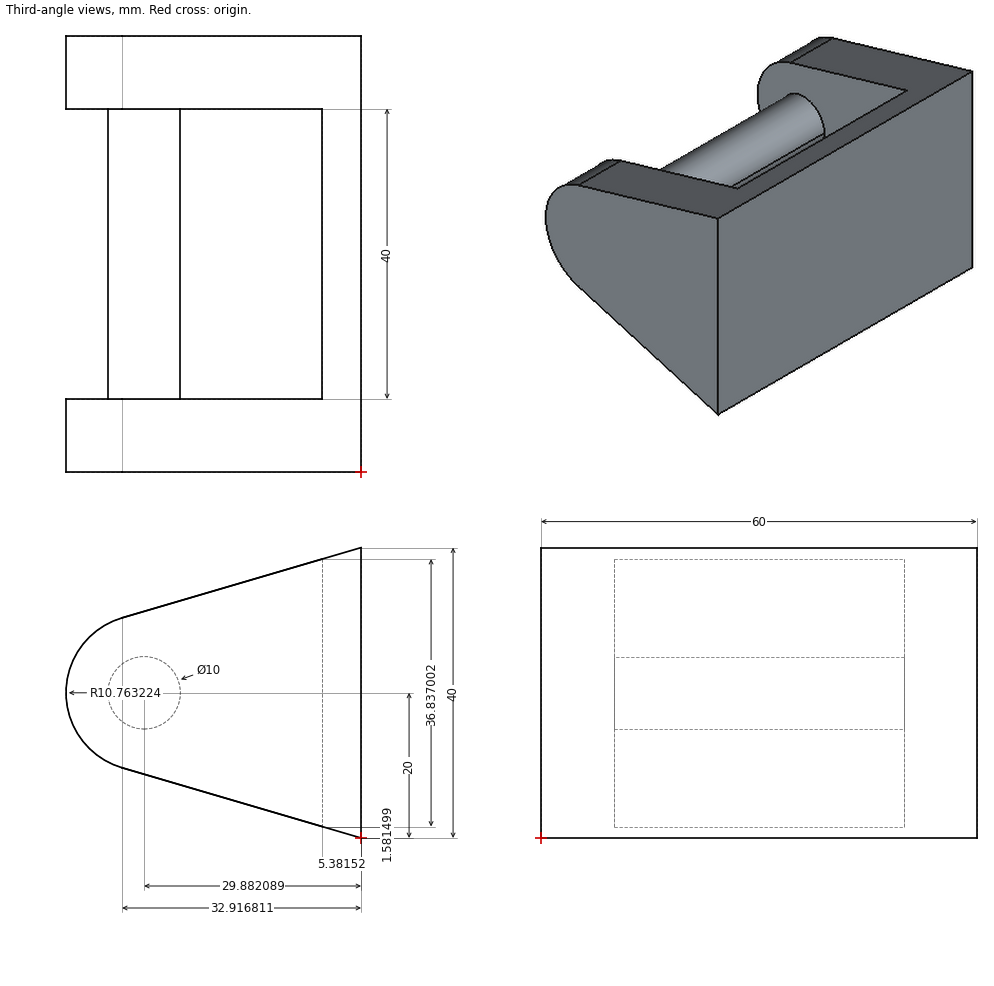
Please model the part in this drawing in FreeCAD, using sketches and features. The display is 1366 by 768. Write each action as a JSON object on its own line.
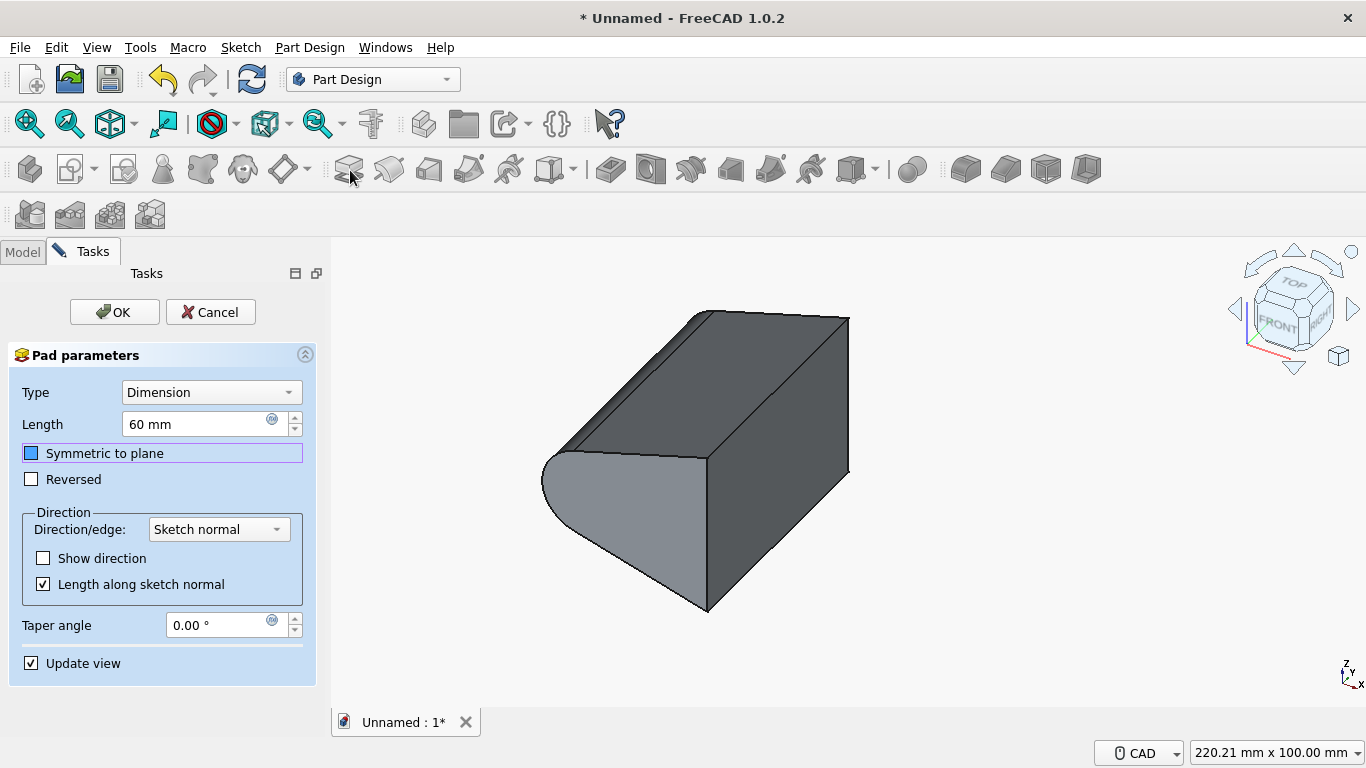
{"action": "left_click", "coordinate": [30, 479]}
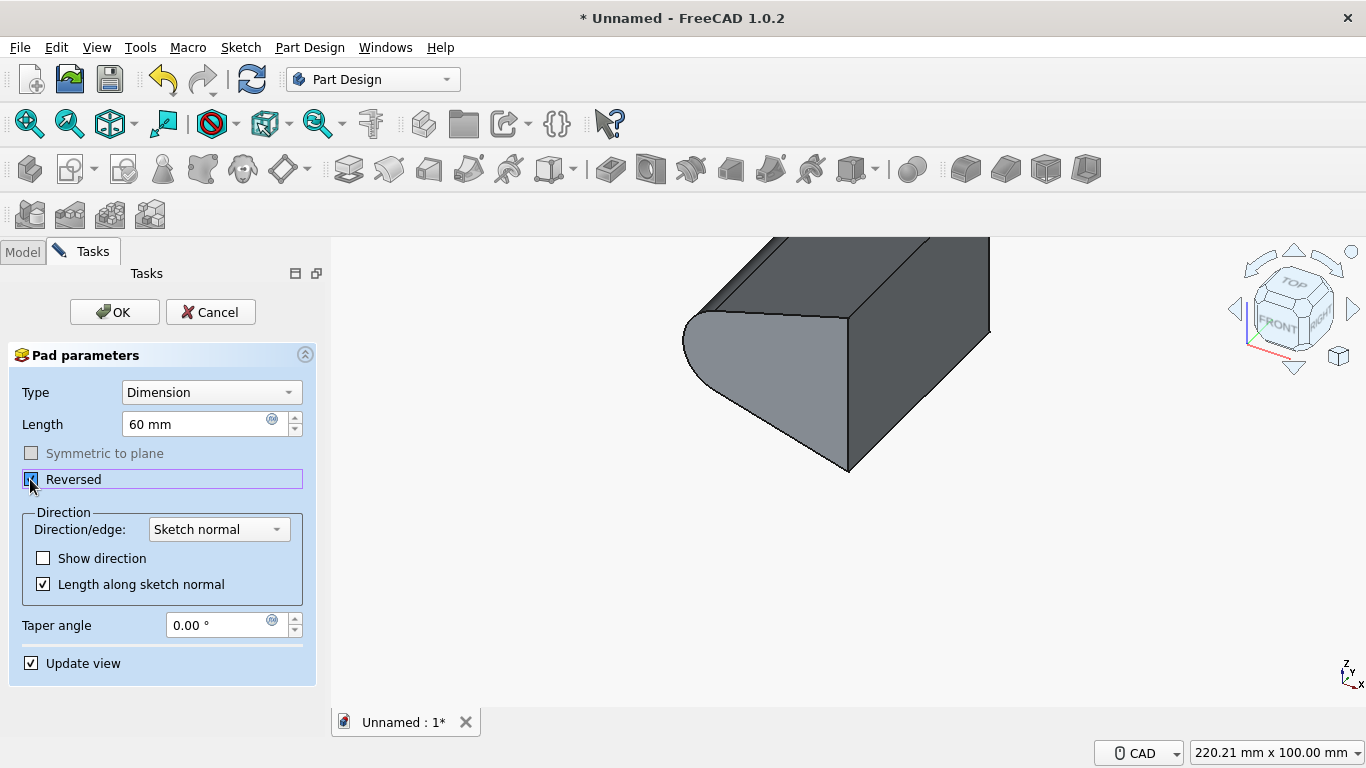
{"action": "left_click", "coordinate": [115, 312]}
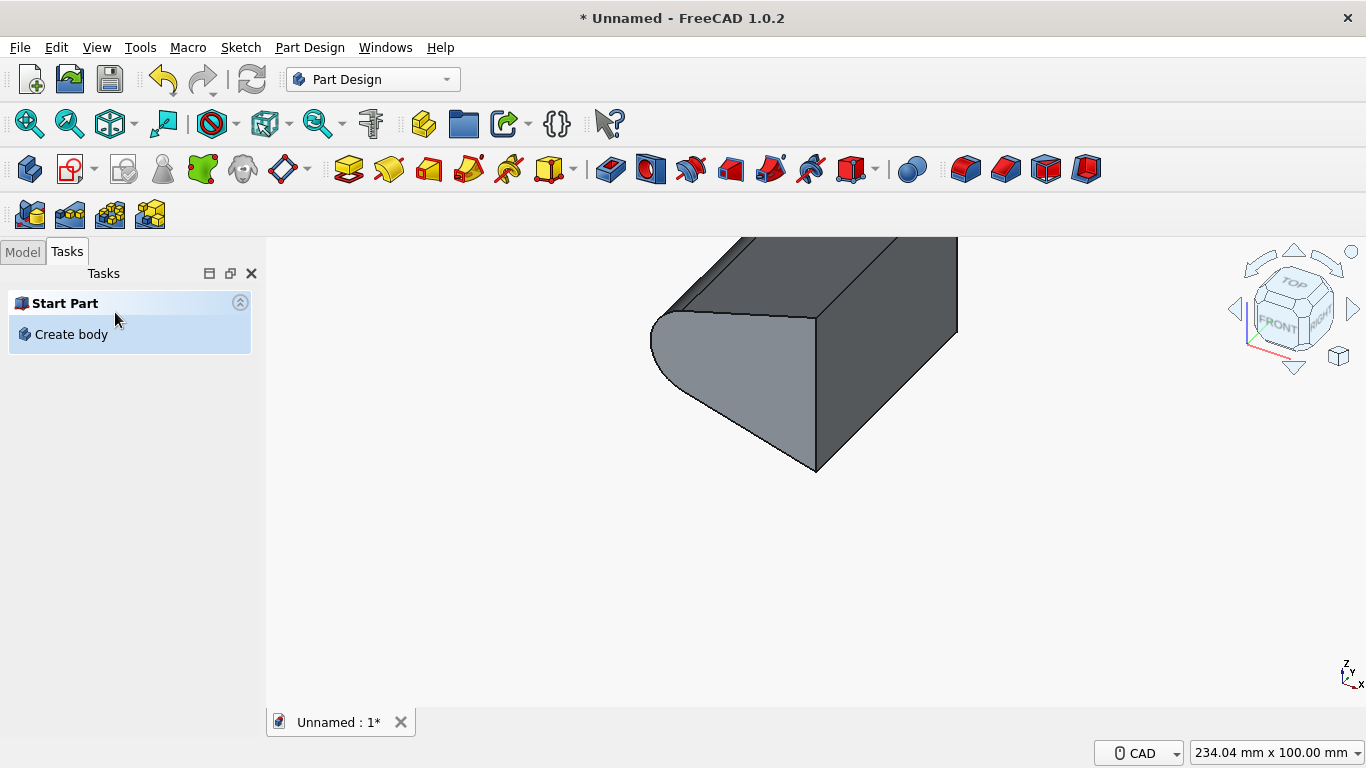
{"action": "left_click", "coordinate": [30, 124]}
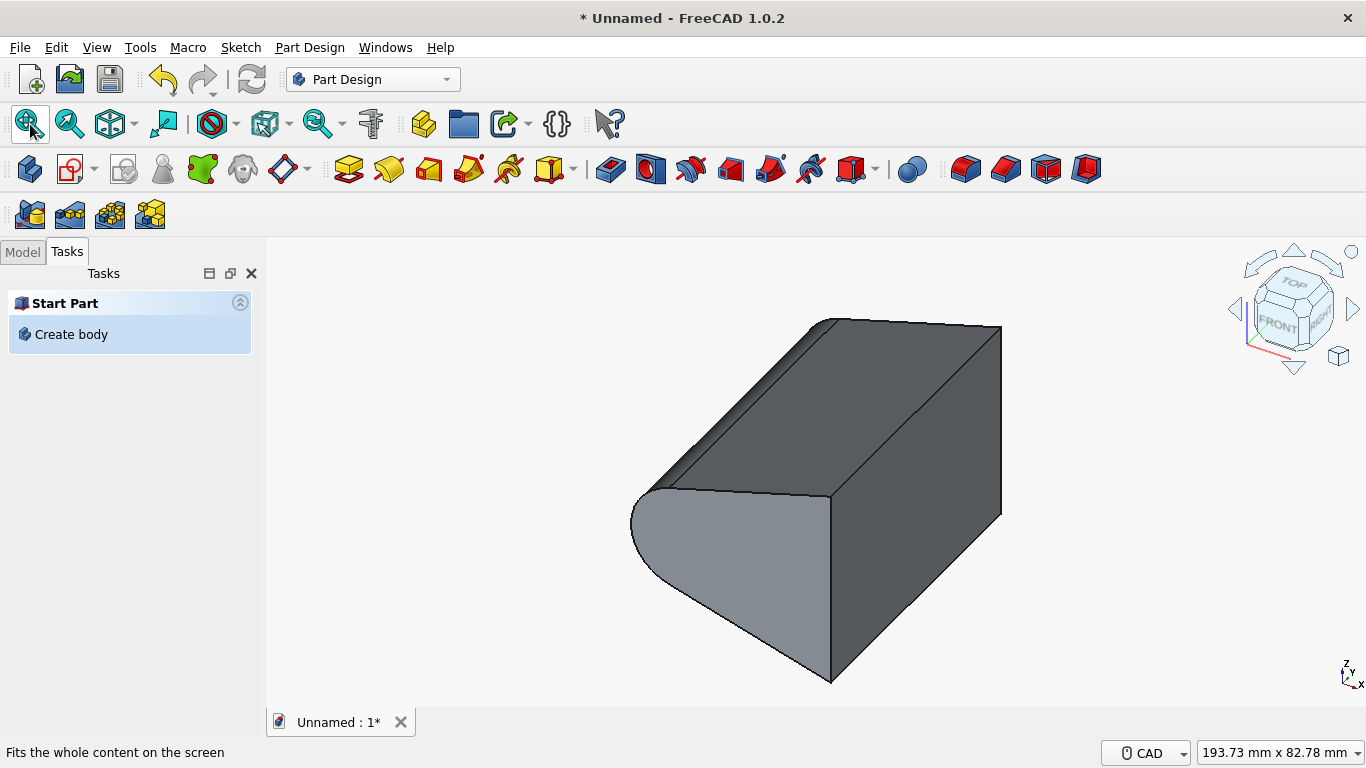
{"action": "left_click", "coordinate": [23, 251]}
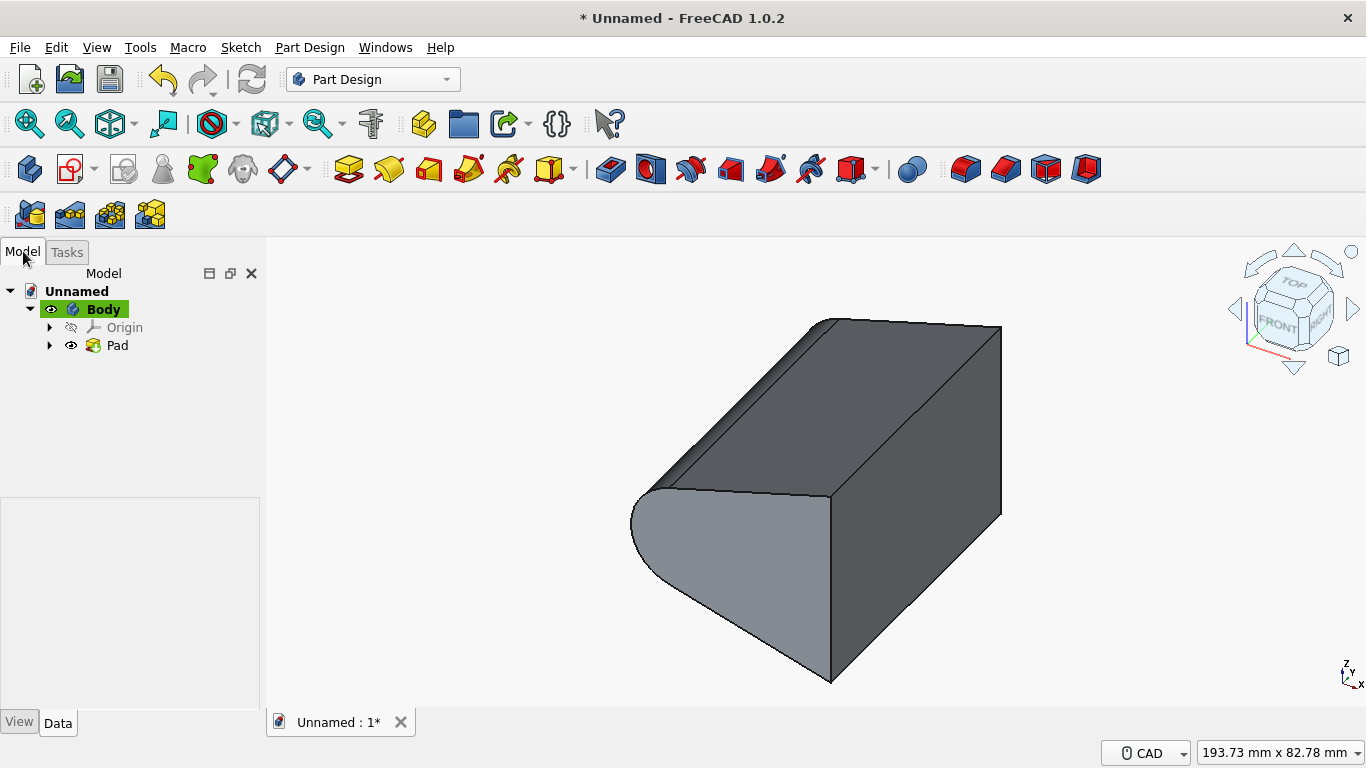
{"action": "left_click", "coordinate": [50, 327]}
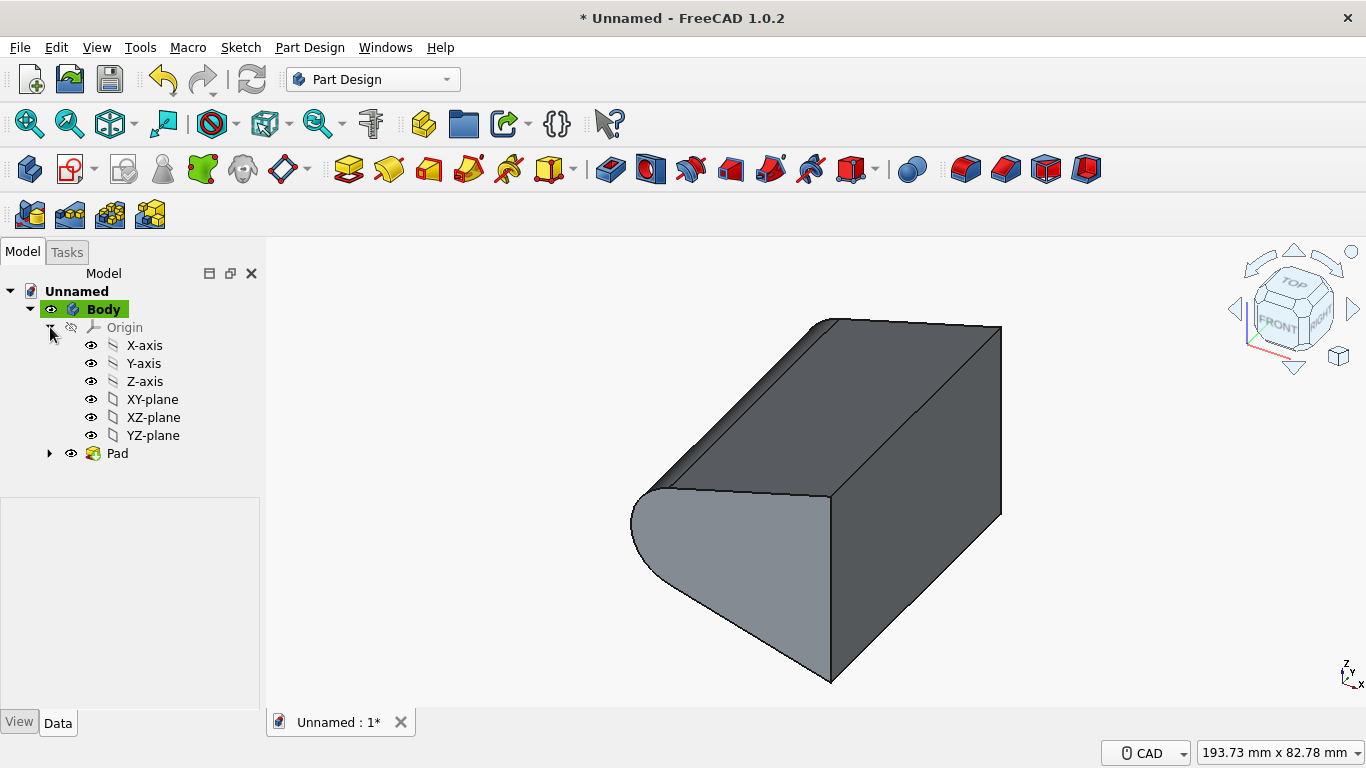
{"action": "left_click", "coordinate": [136, 417]}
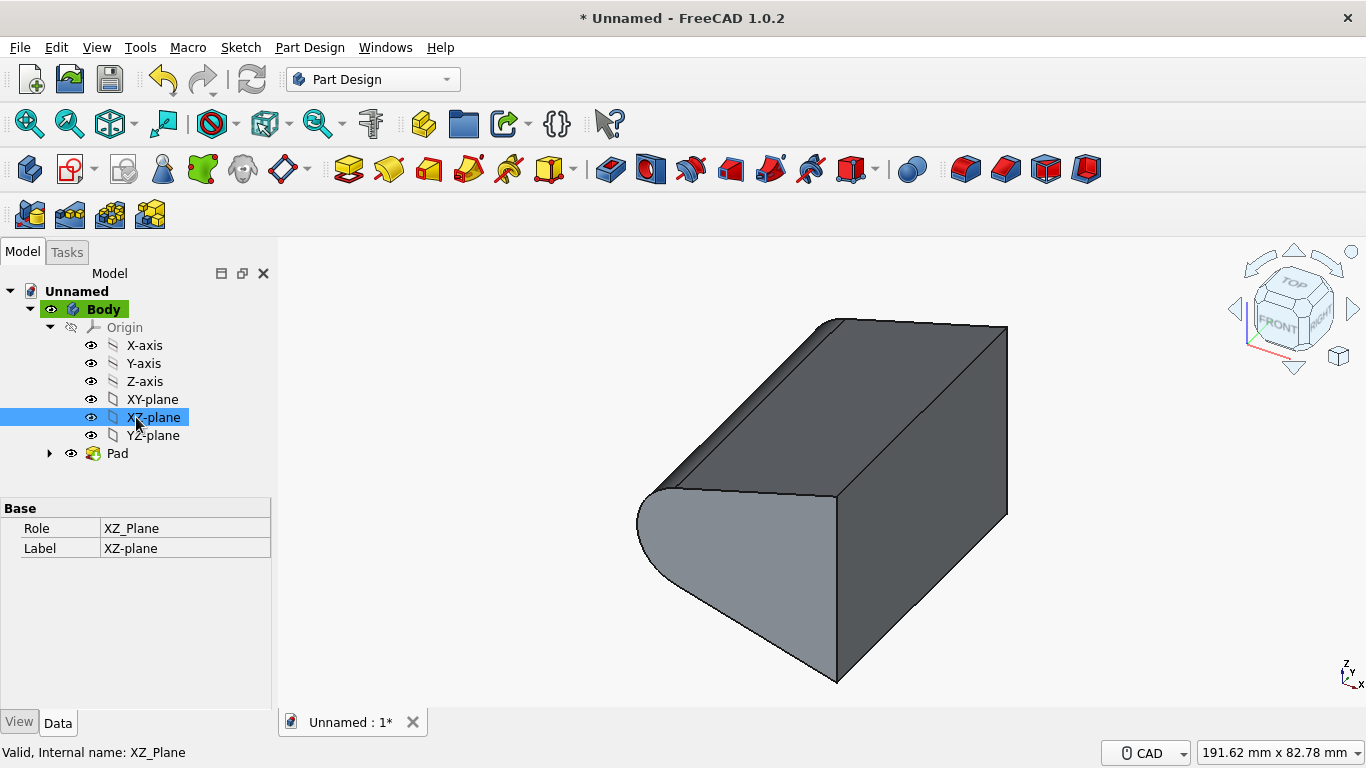
{"action": "left_click", "coordinate": [284, 170]}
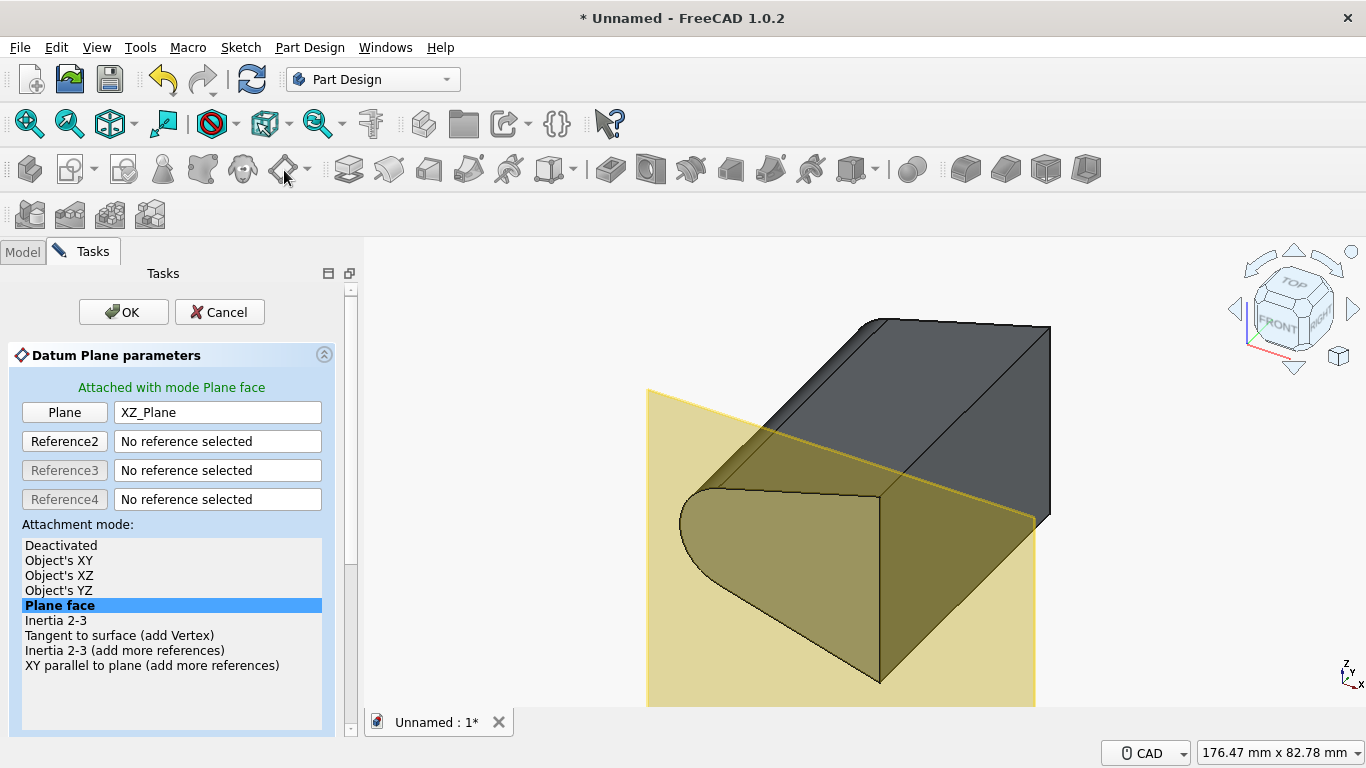
{"action": "scroll", "coordinate": [351, 510], "scroll_direction": "down", "scroll_amount": 3}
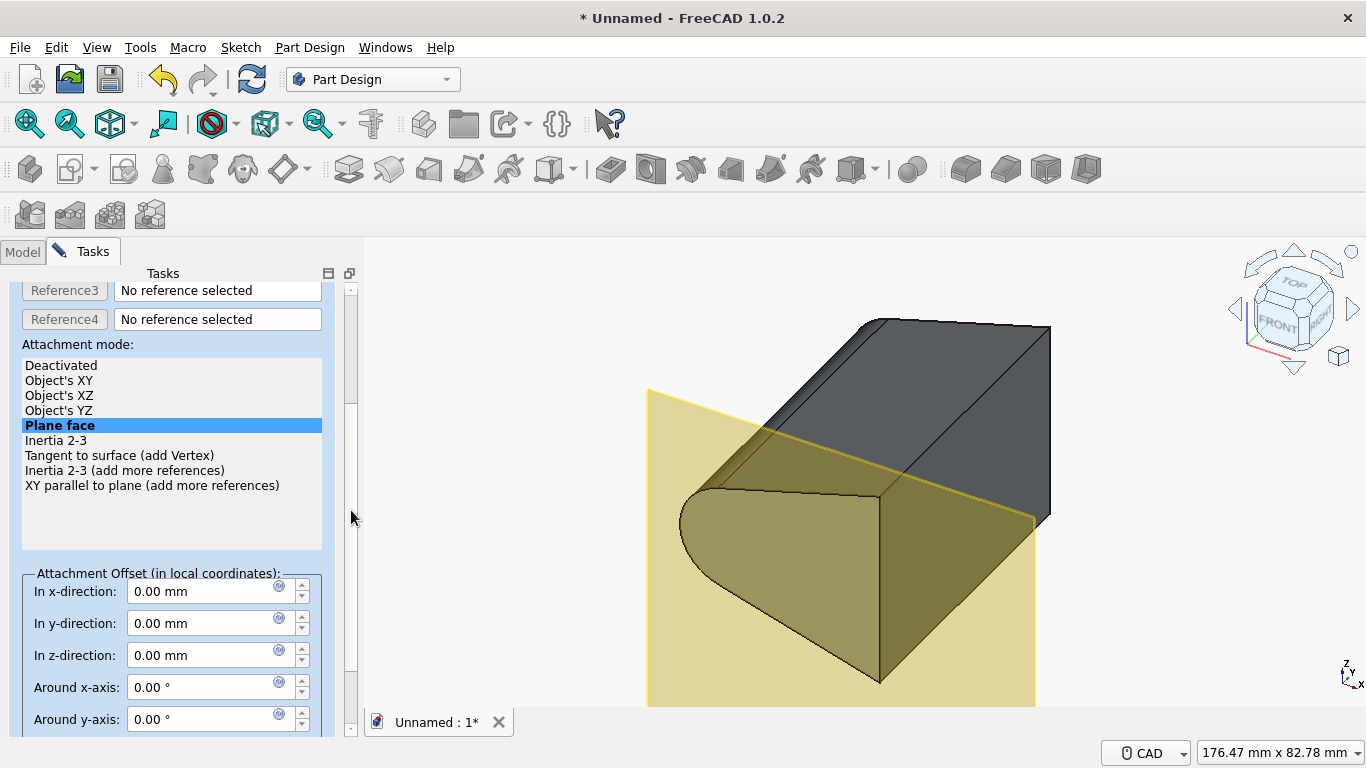
{"action": "triple_click", "coordinate": [210, 655]}